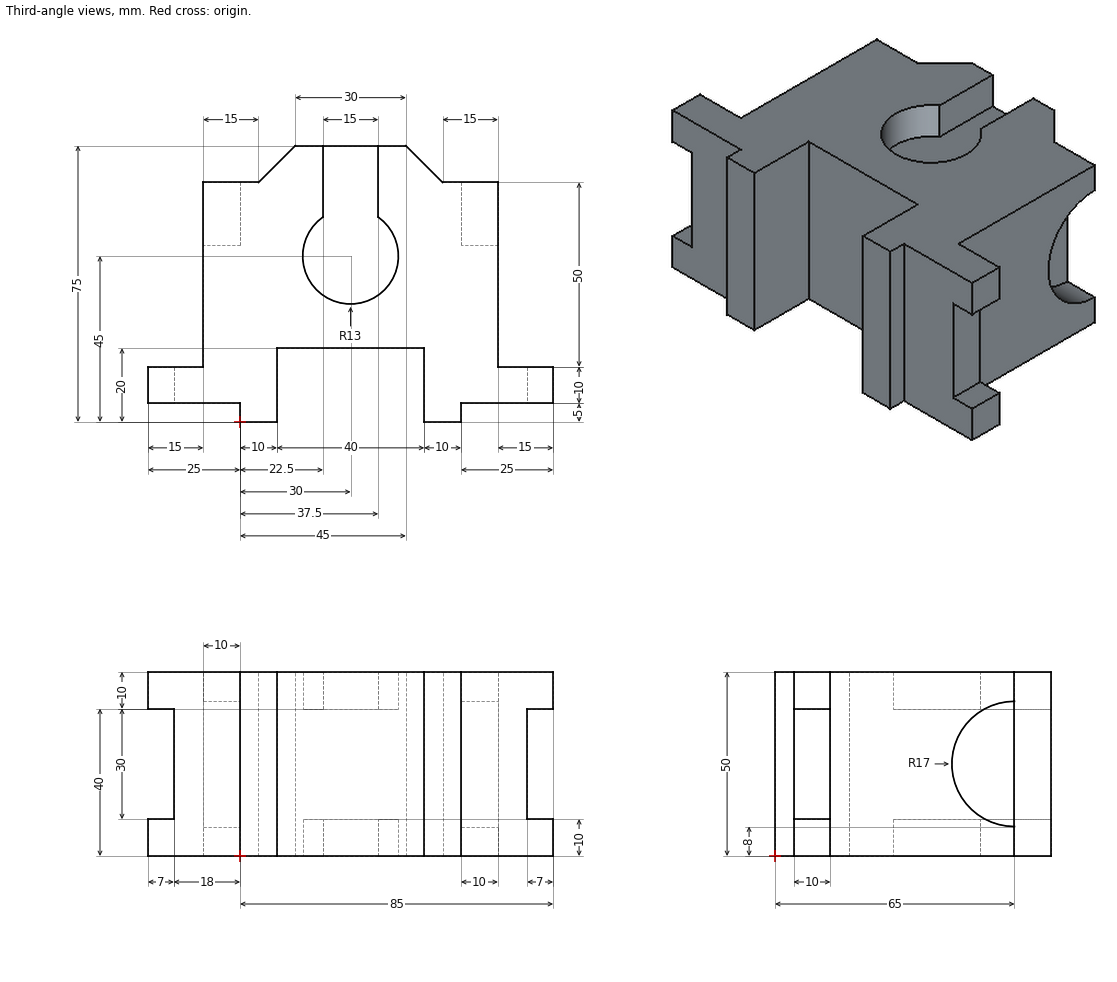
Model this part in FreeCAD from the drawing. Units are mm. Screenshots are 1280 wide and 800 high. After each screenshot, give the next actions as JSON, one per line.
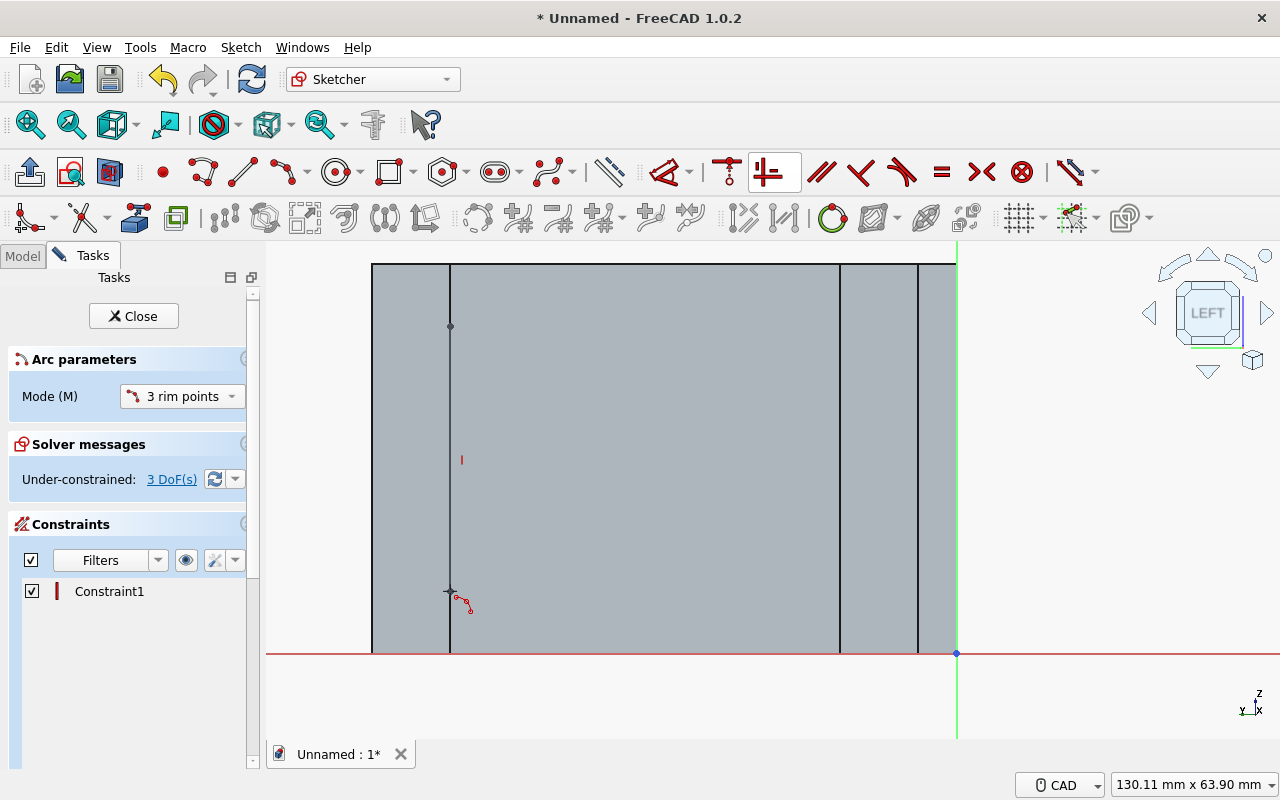
{"action": "left_click", "coordinate": [450, 592]}
{"action": "left_click", "coordinate": [450, 327]}
{"action": "left_click", "coordinate": [583, 459]}
{"action": "key", "text": "Escape"}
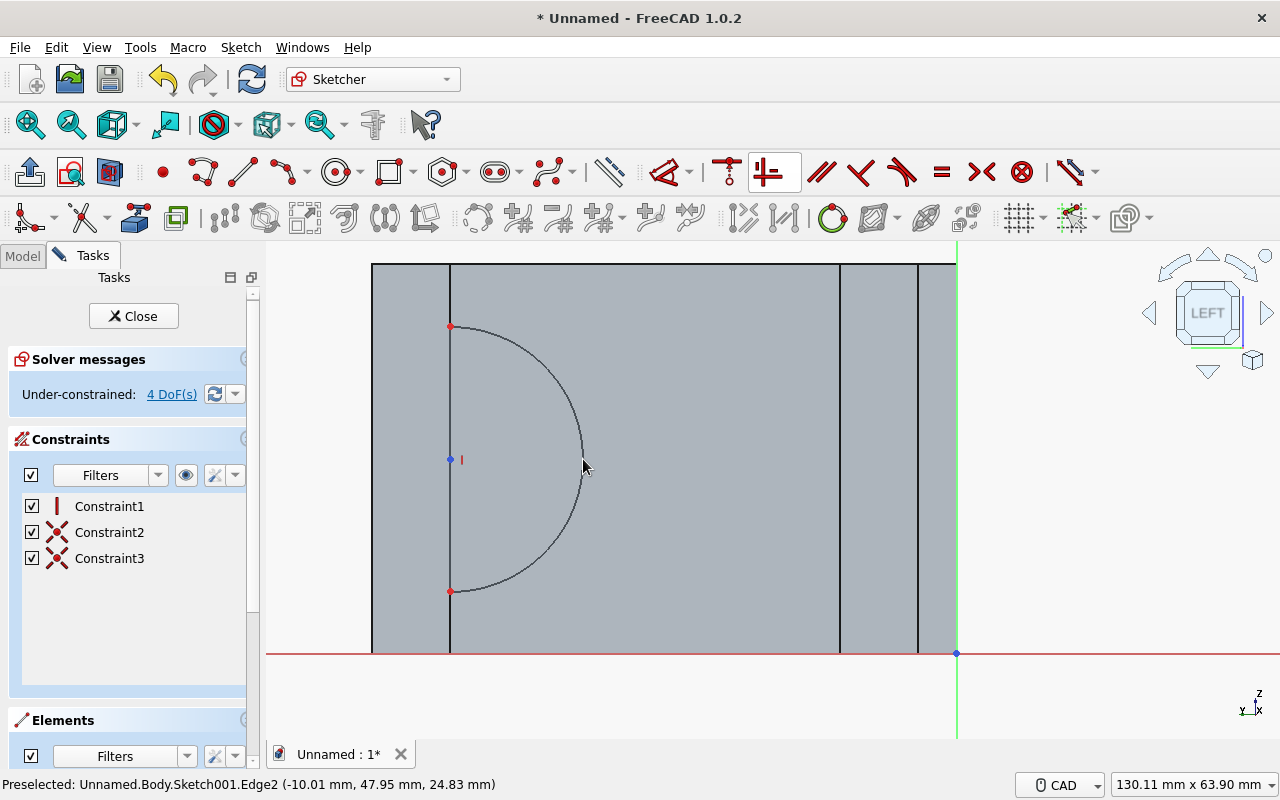
{"action": "key", "text": "d"}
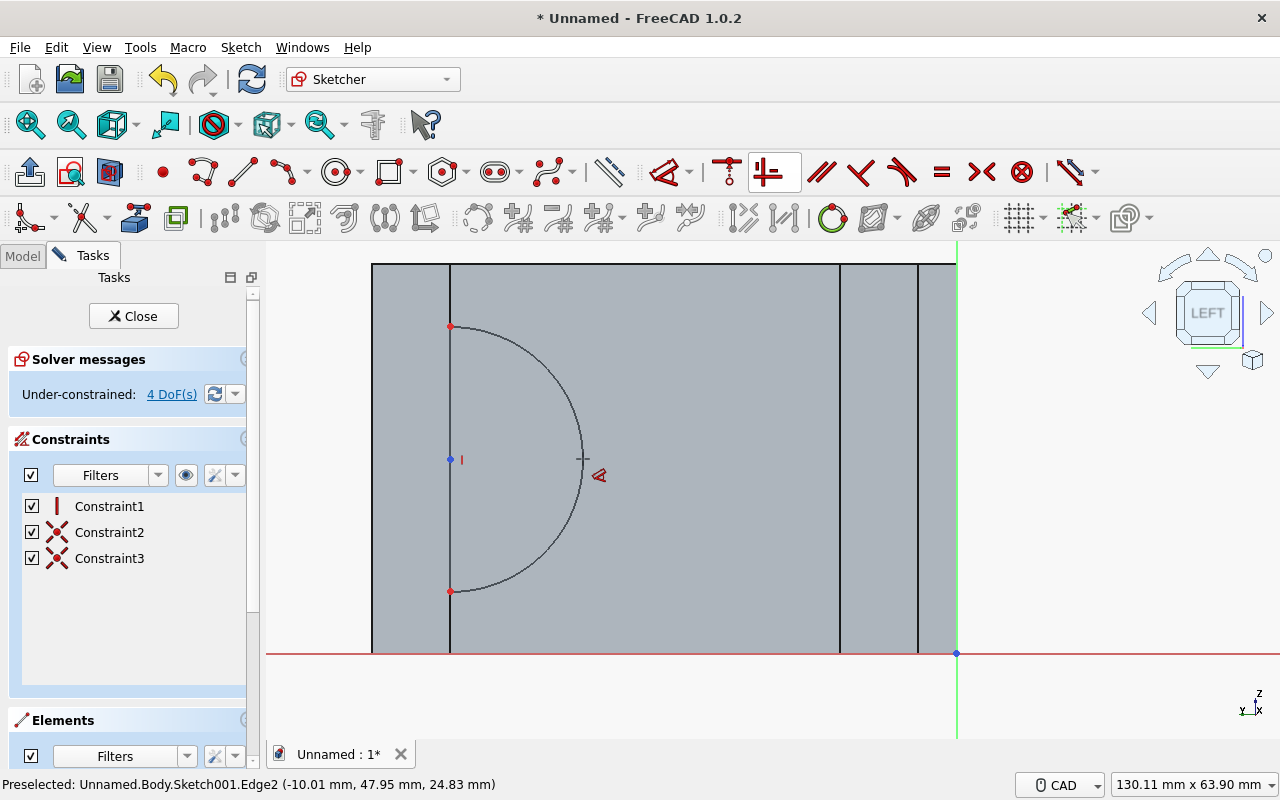
{"action": "left_click", "coordinate": [558, 538]}
{"action": "left_click", "coordinate": [584, 557]}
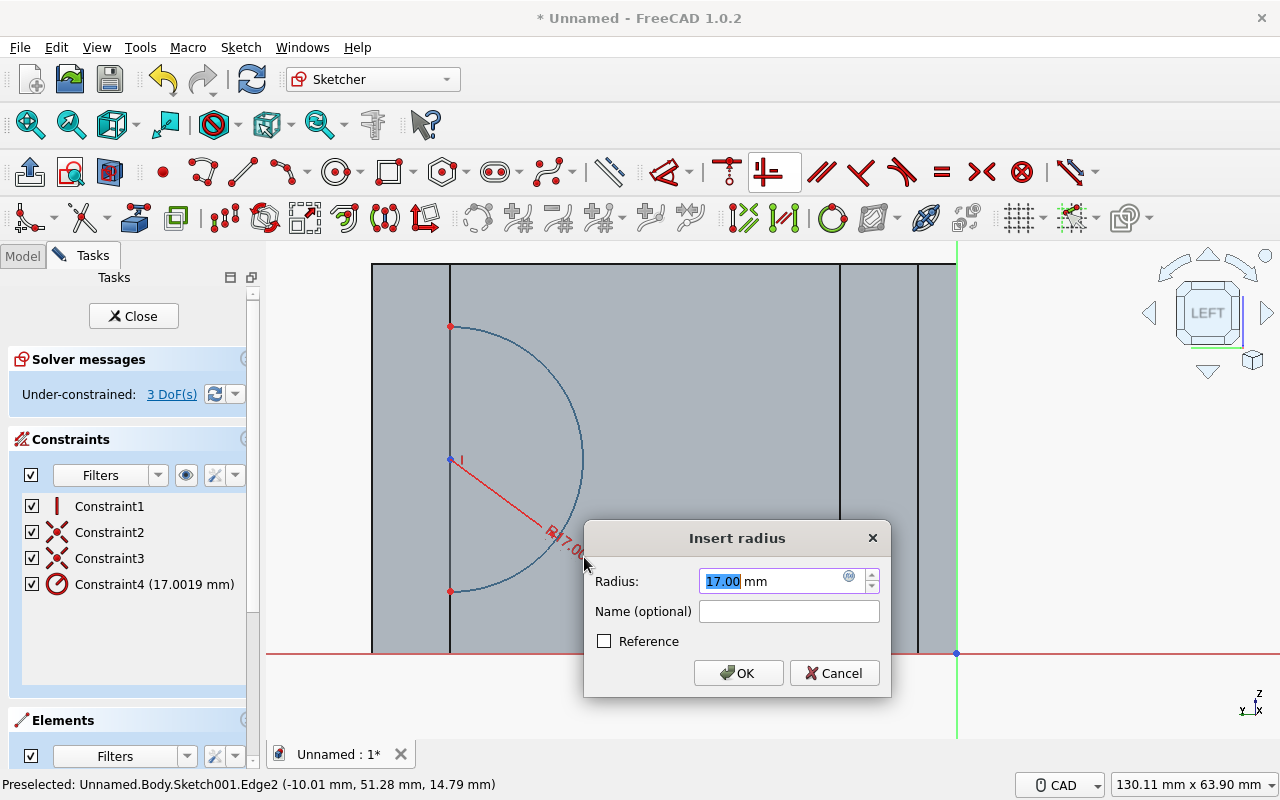
{"action": "type", "text": "17"}
{"action": "key", "text": "Return"}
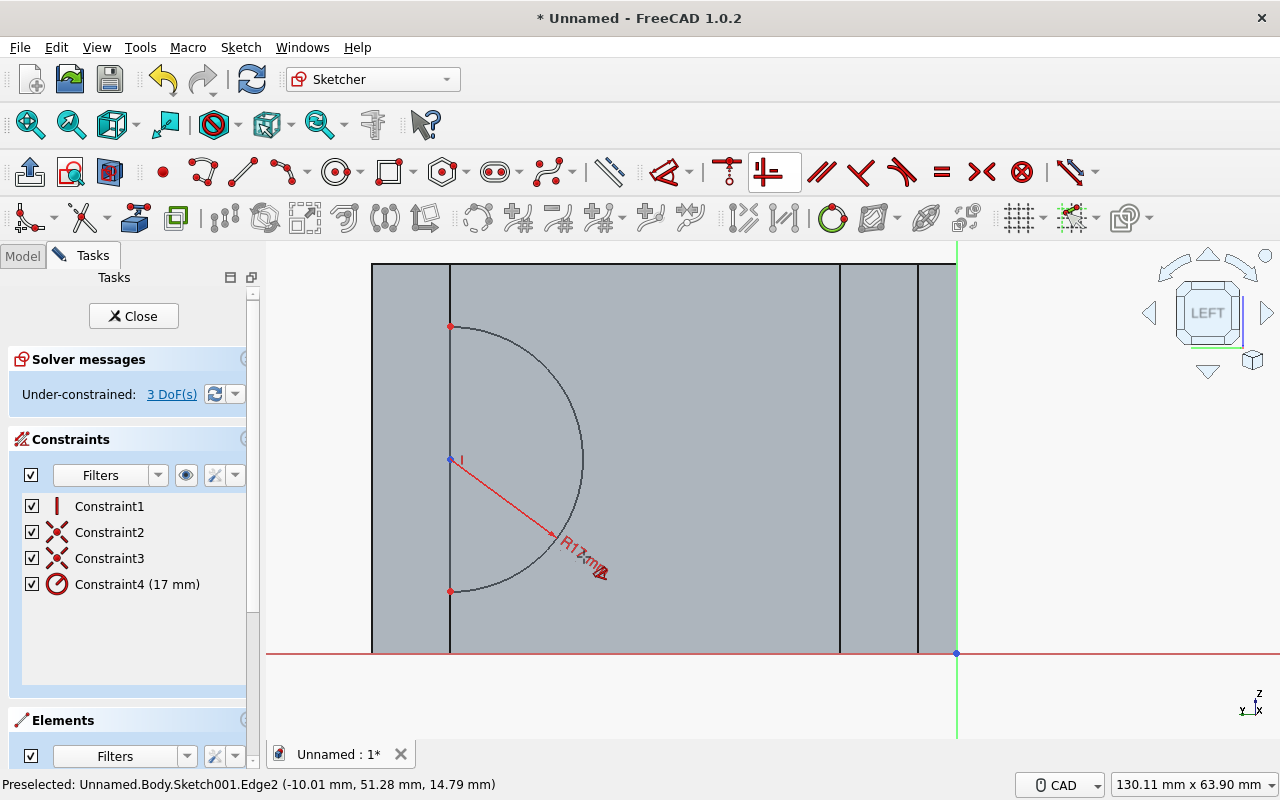
{"action": "left_click", "coordinate": [450, 592]}
{"action": "left_click", "coordinate": [416, 623]}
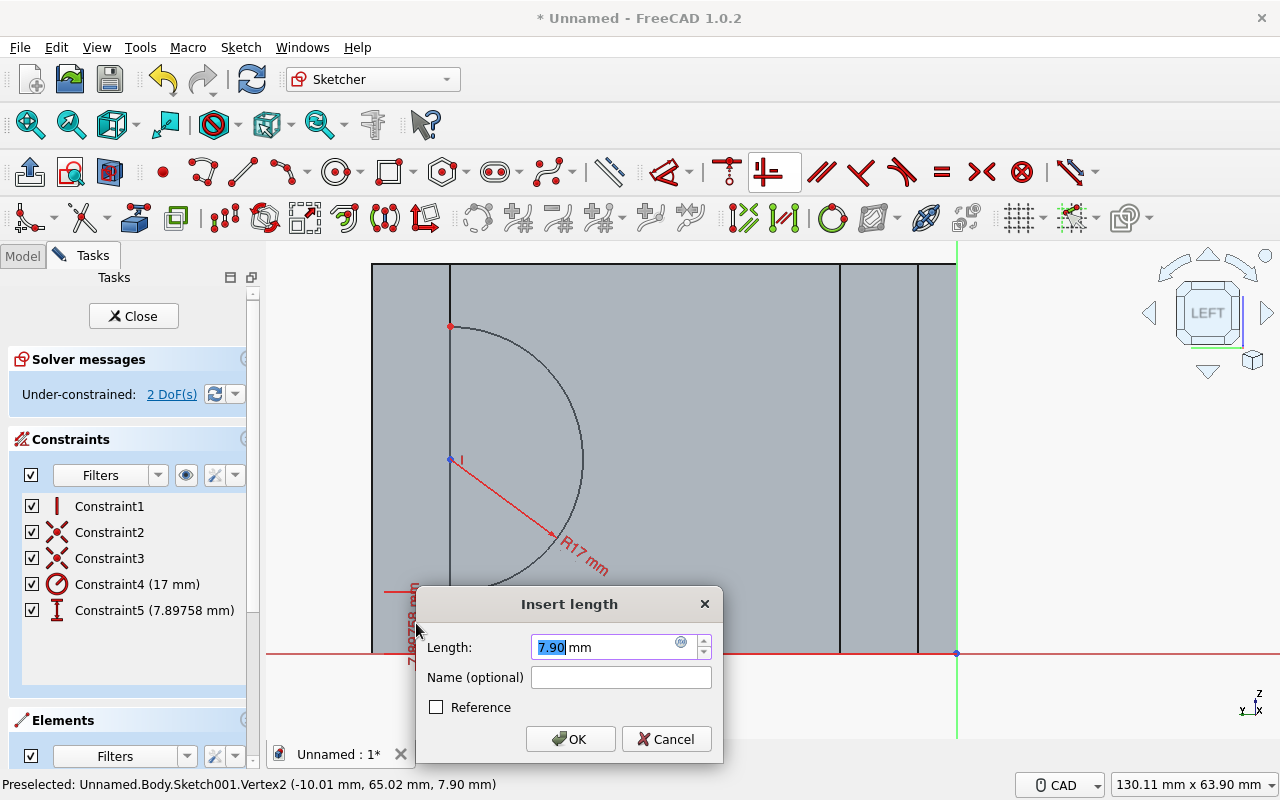
{"action": "type", "text": "8"}
{"action": "key", "text": "Return"}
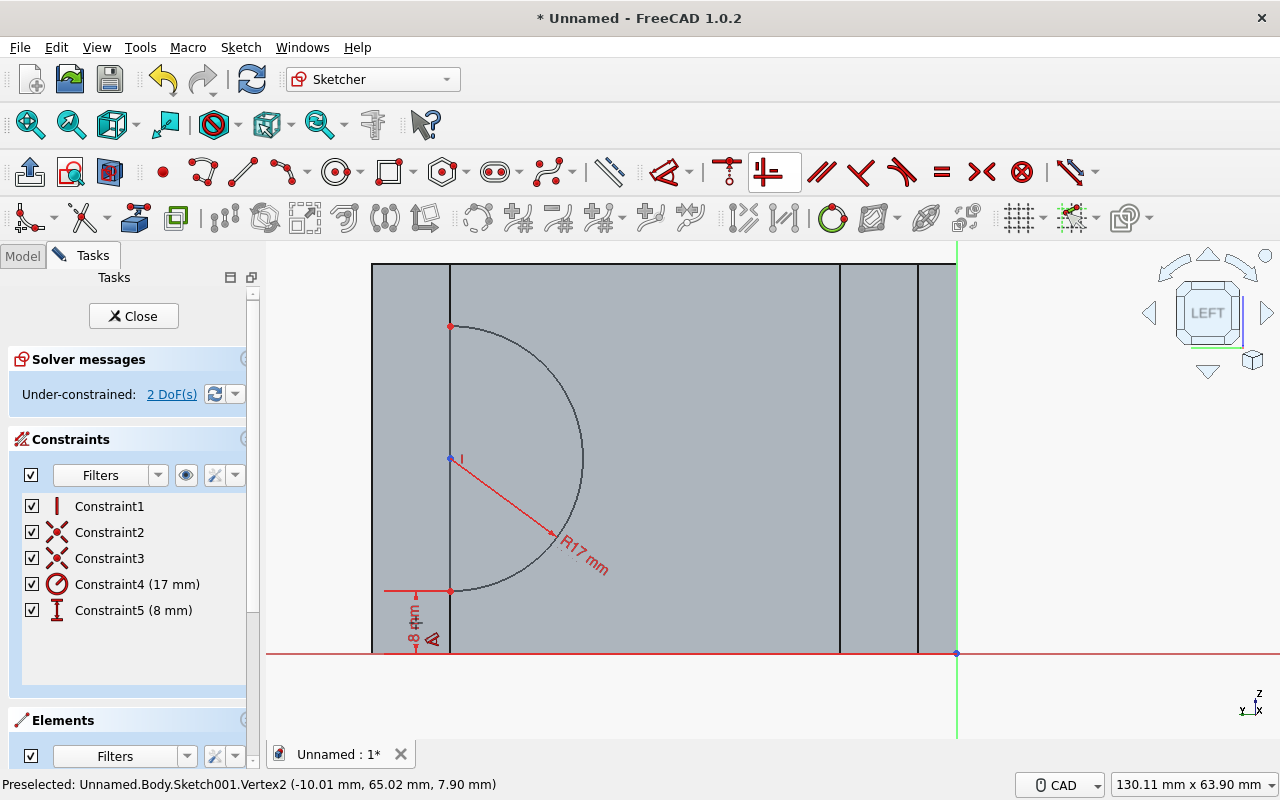
{"action": "left_click", "coordinate": [450, 326]}
{"action": "left_click", "coordinate": [703, 688]}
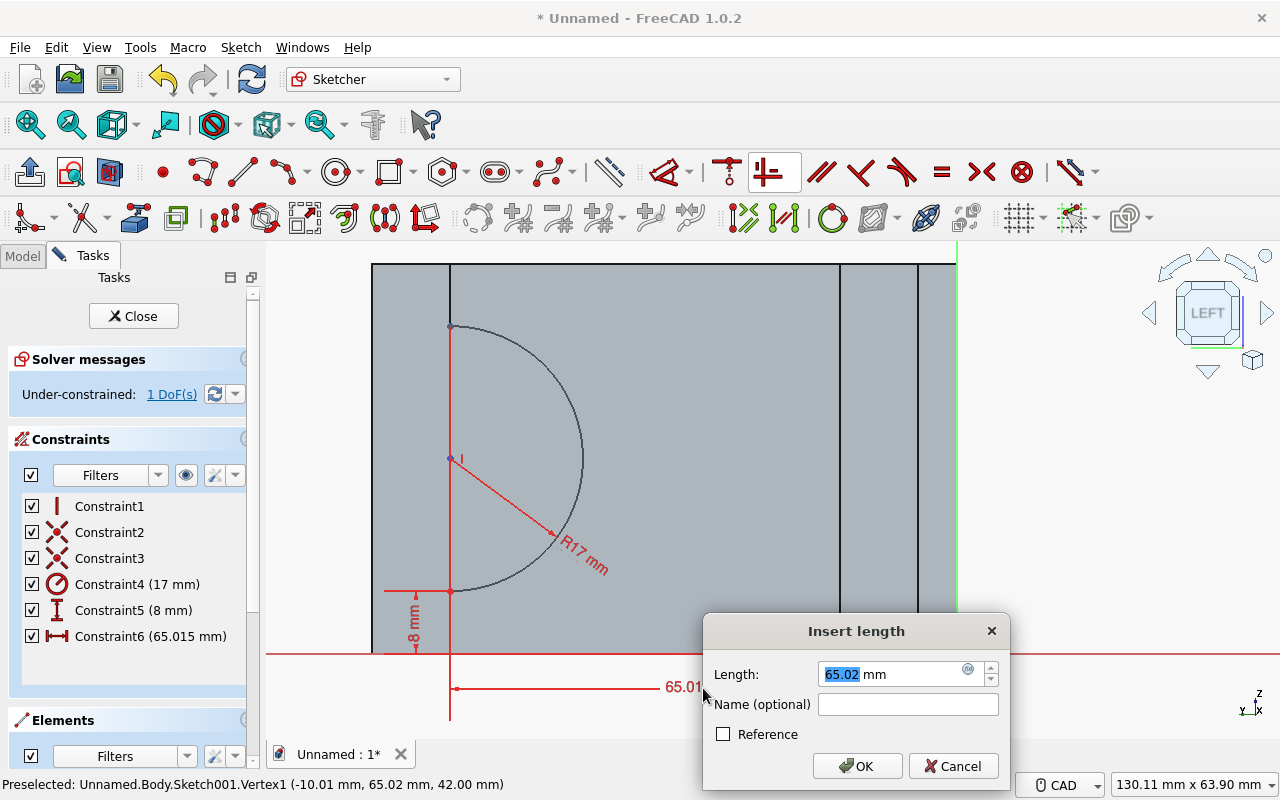
{"action": "type", "text": "65"}
{"action": "key", "text": "Return"}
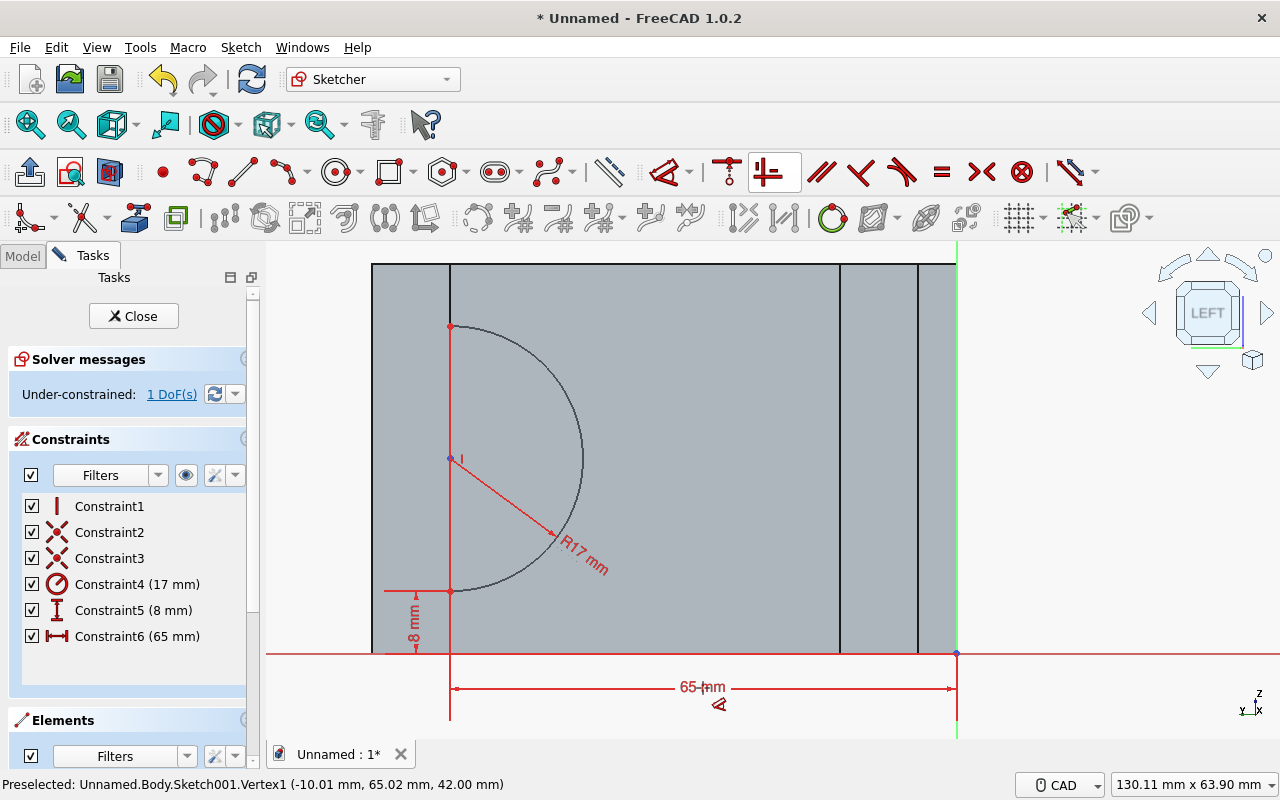
{"action": "left_click", "coordinate": [451, 459]}
{"action": "left_click", "coordinate": [587, 688]}